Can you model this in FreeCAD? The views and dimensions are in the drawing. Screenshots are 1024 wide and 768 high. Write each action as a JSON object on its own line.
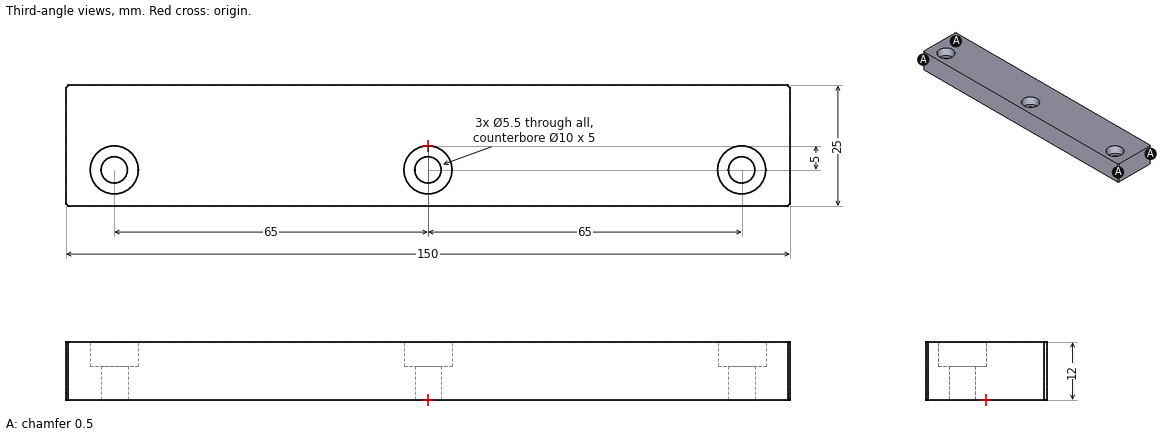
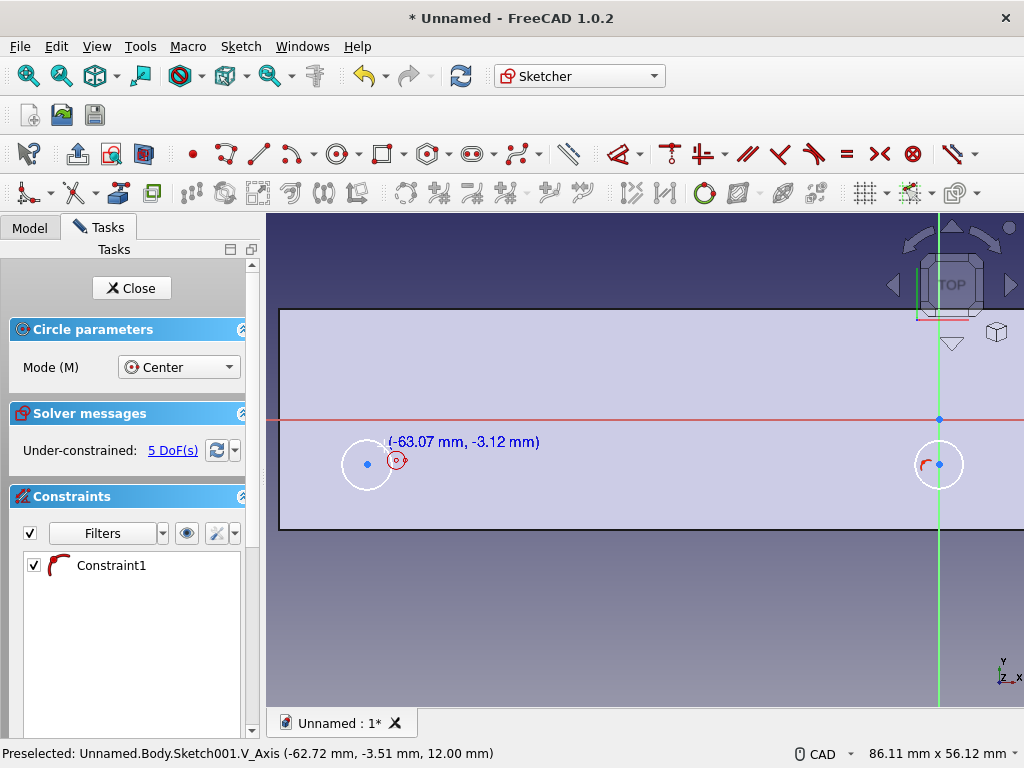
{"action": "scroll", "coordinate": [365, 464], "scroll_direction": "down", "scroll_amount": 5}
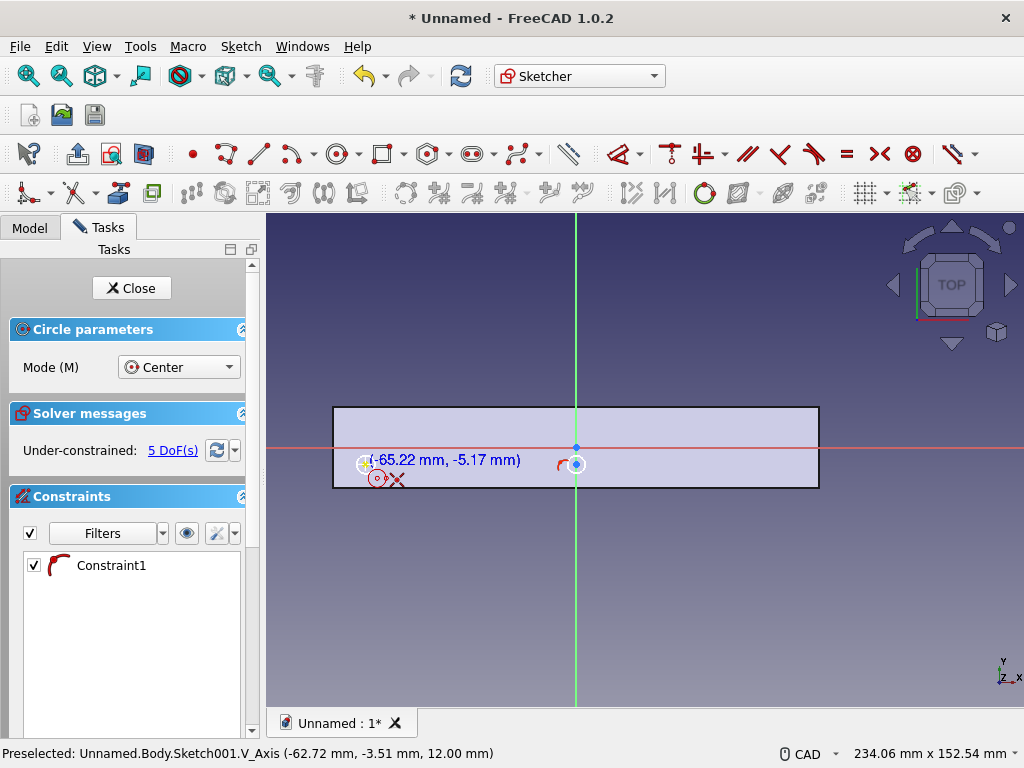
{"action": "scroll", "coordinate": [787, 464], "scroll_direction": "up", "scroll_amount": 5}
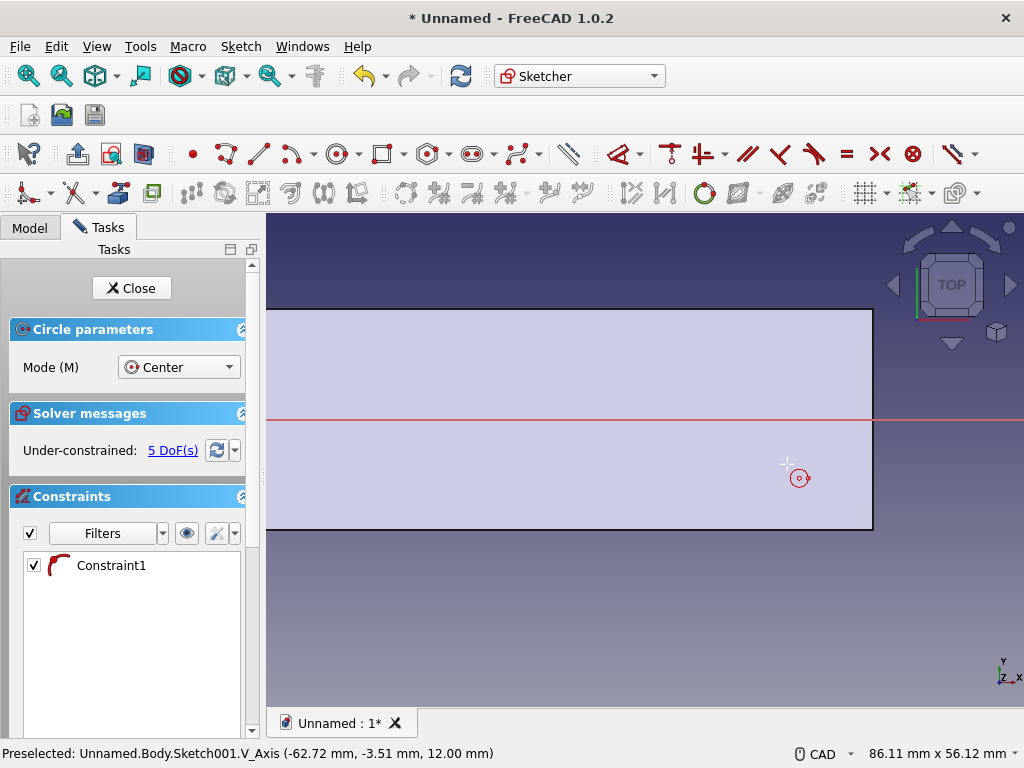
{"action": "left_click", "coordinate": [785, 464]}
{"action": "left_click", "coordinate": [802, 446]}
{"action": "key", "text": "Escape"}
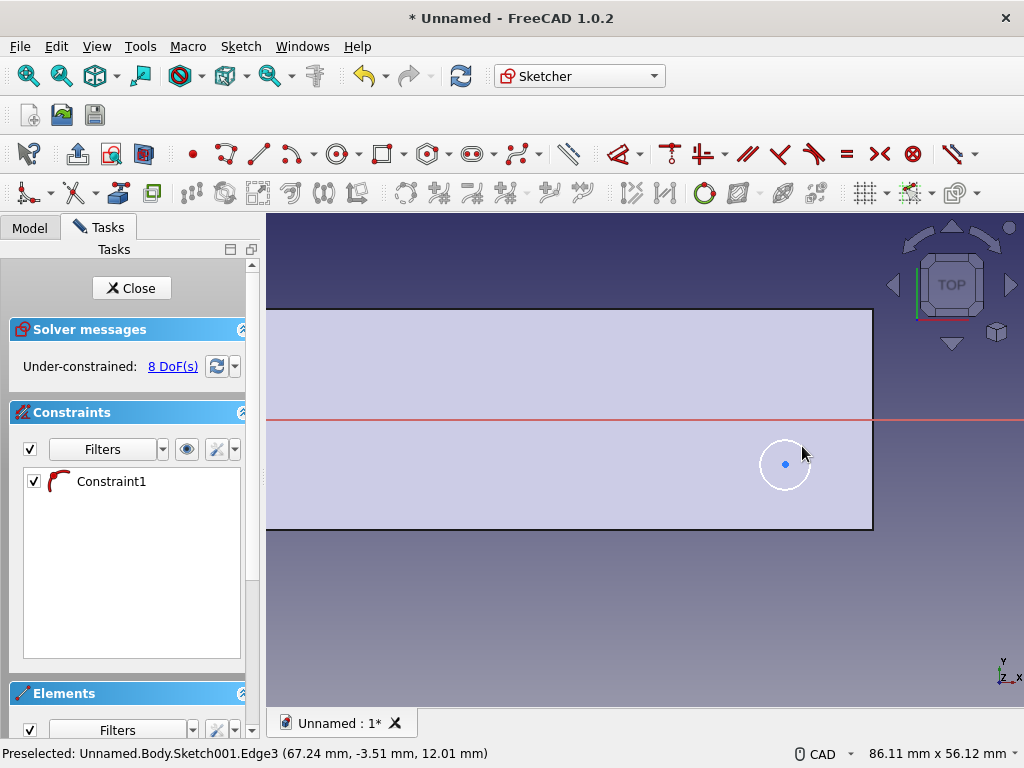
{"action": "scroll", "coordinate": [788, 464], "scroll_direction": "down", "scroll_amount": 5}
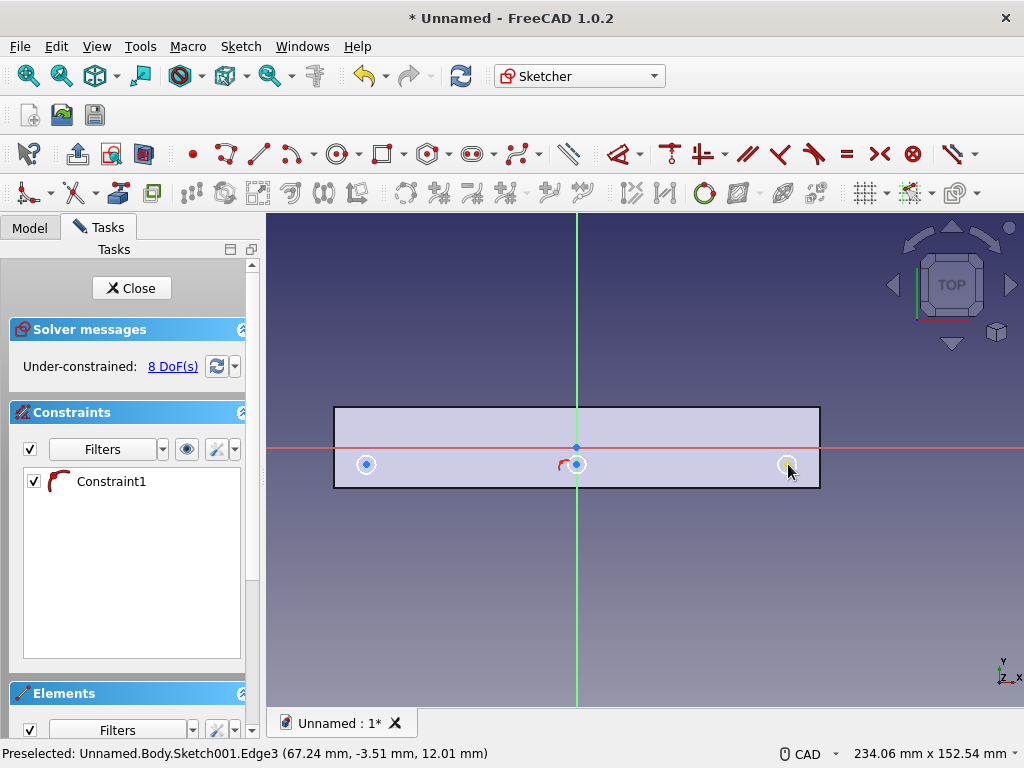
{"action": "scroll", "coordinate": [583, 458], "scroll_direction": "up", "scroll_amount": 5}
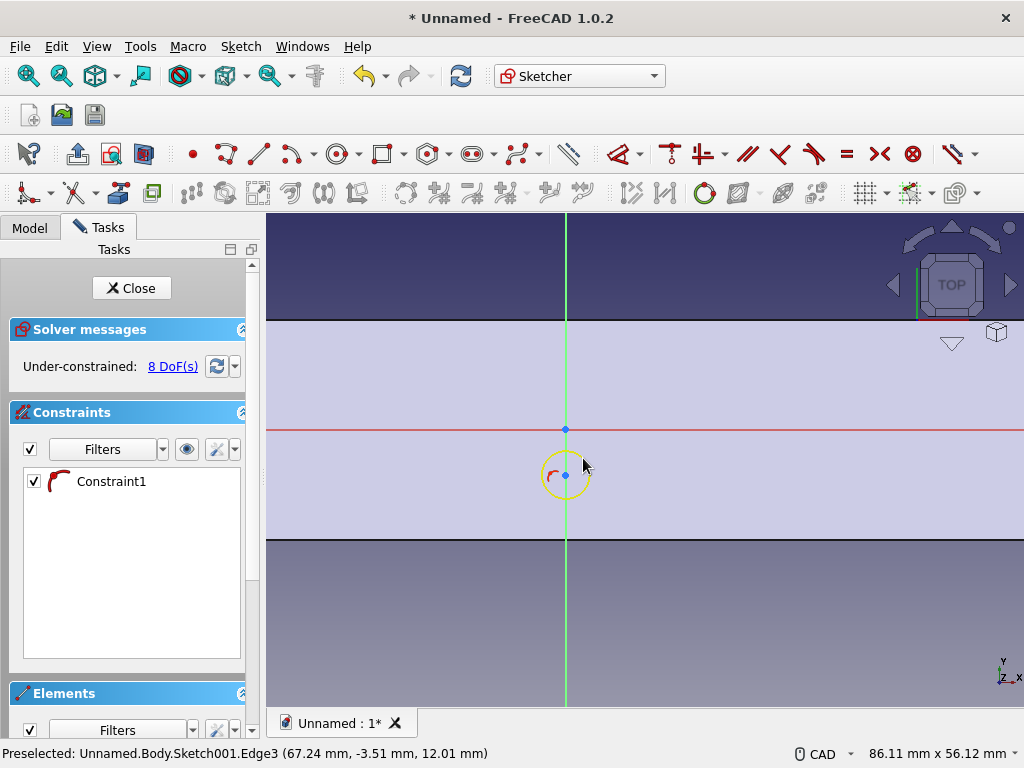
{"action": "left_click", "coordinate": [583, 458]}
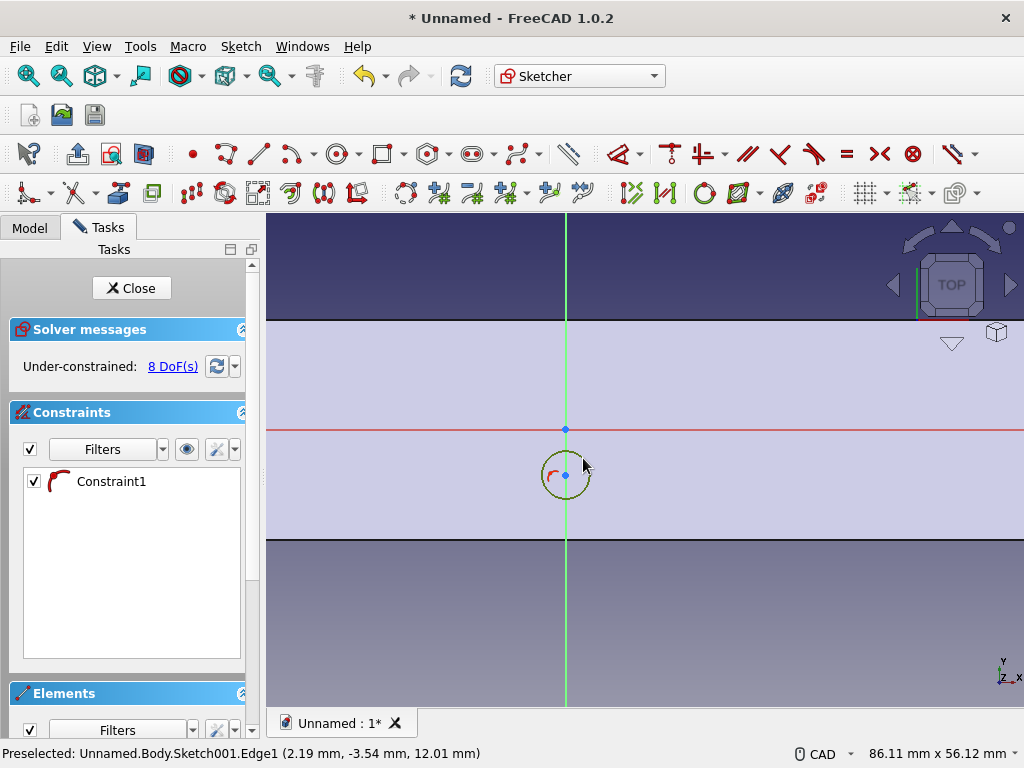
{"action": "scroll", "coordinate": [583, 458], "scroll_direction": "down", "scroll_amount": 5}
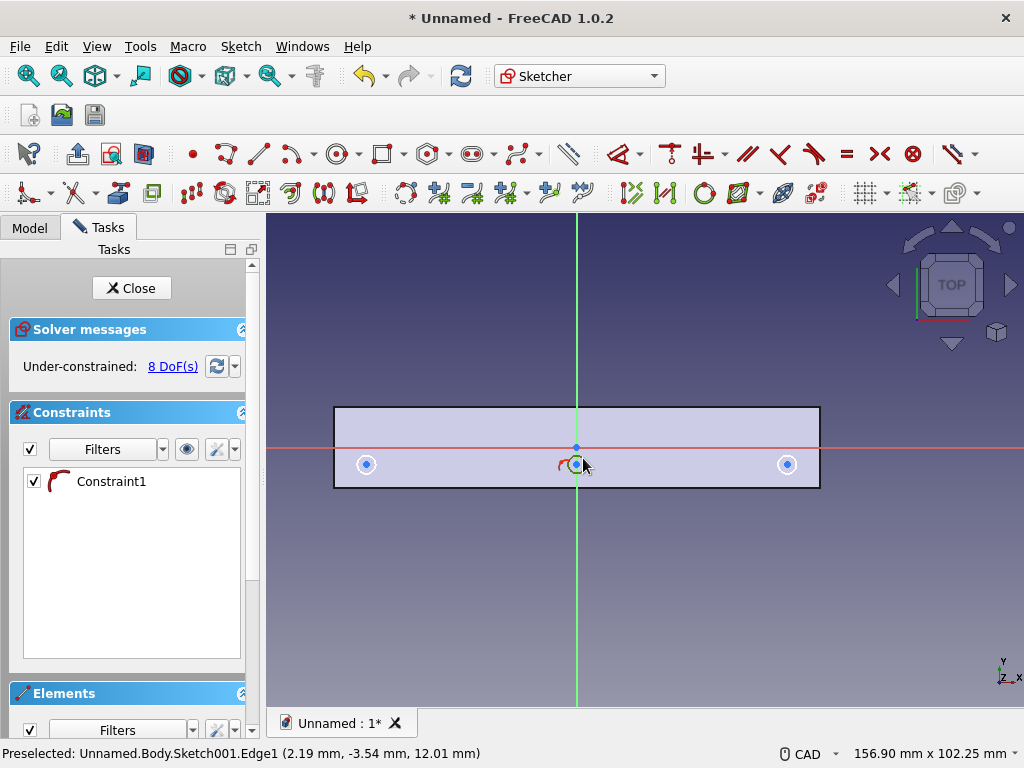
{"action": "scroll", "coordinate": [373, 458], "scroll_direction": "up", "scroll_amount": 3}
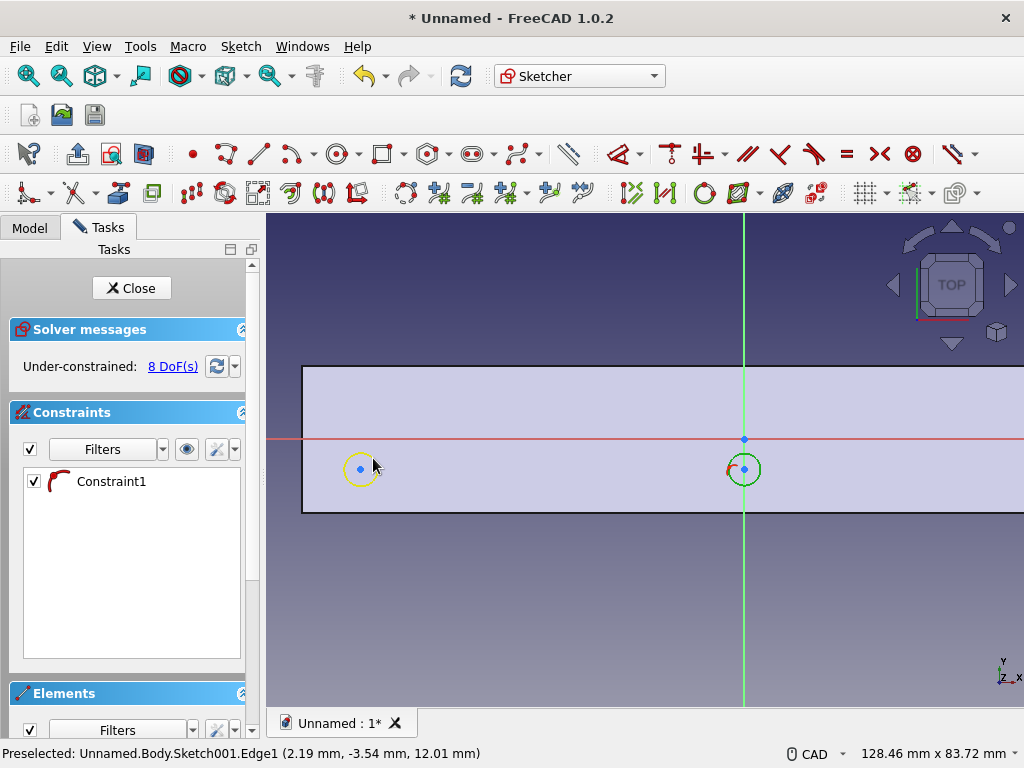
{"action": "left_click", "coordinate": [373, 458]}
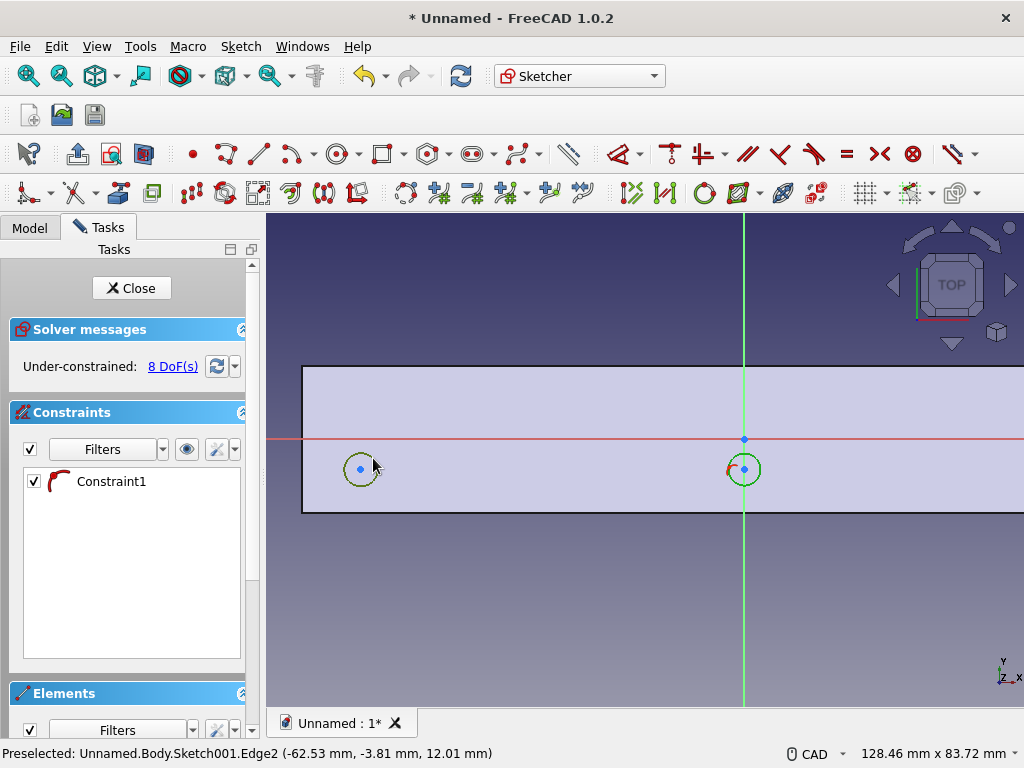
{"action": "scroll", "coordinate": [372, 457], "scroll_direction": "down", "scroll_amount": 3}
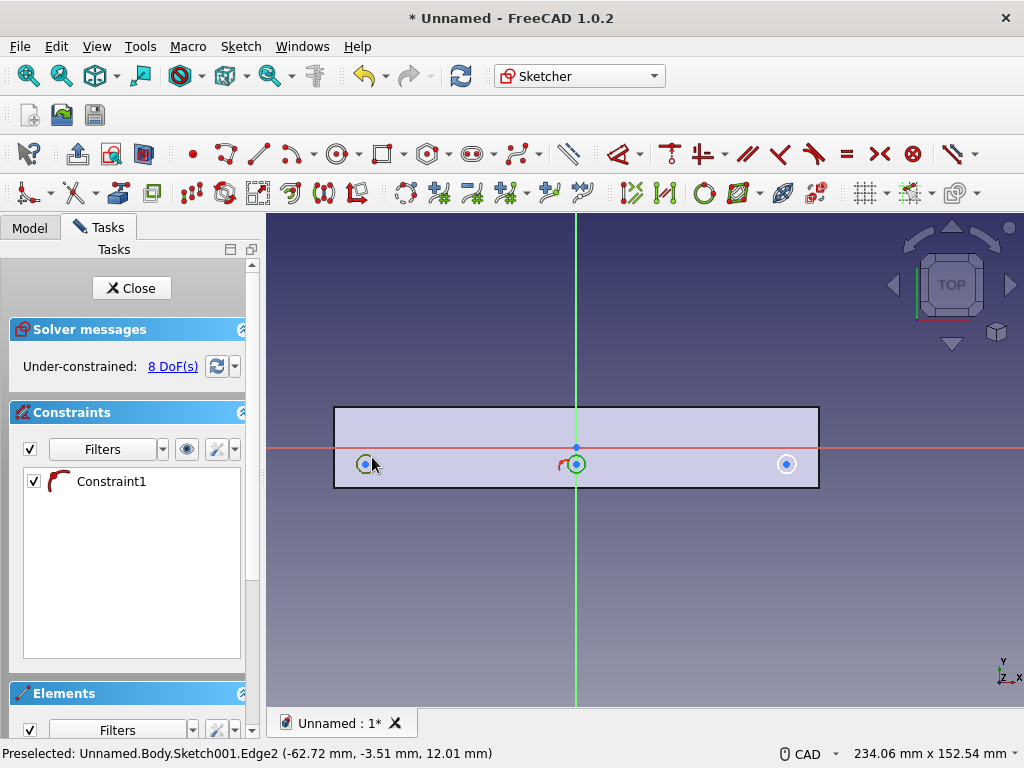
{"action": "scroll", "coordinate": [793, 458], "scroll_direction": "up", "scroll_amount": 3}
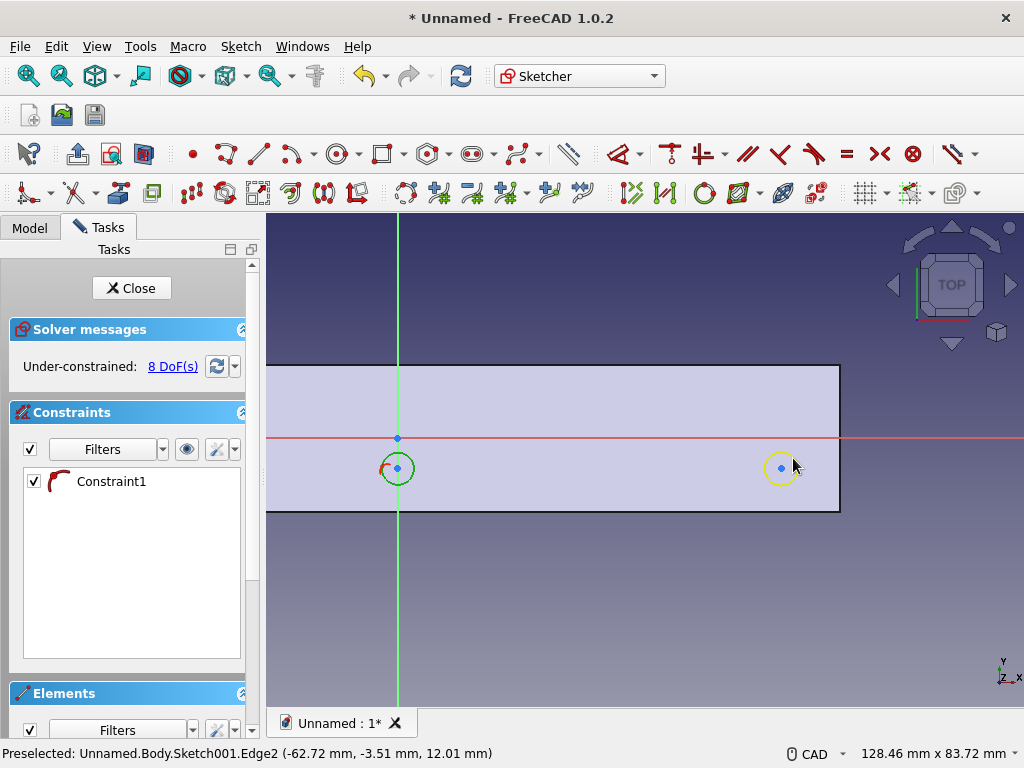
{"action": "left_click", "coordinate": [793, 457]}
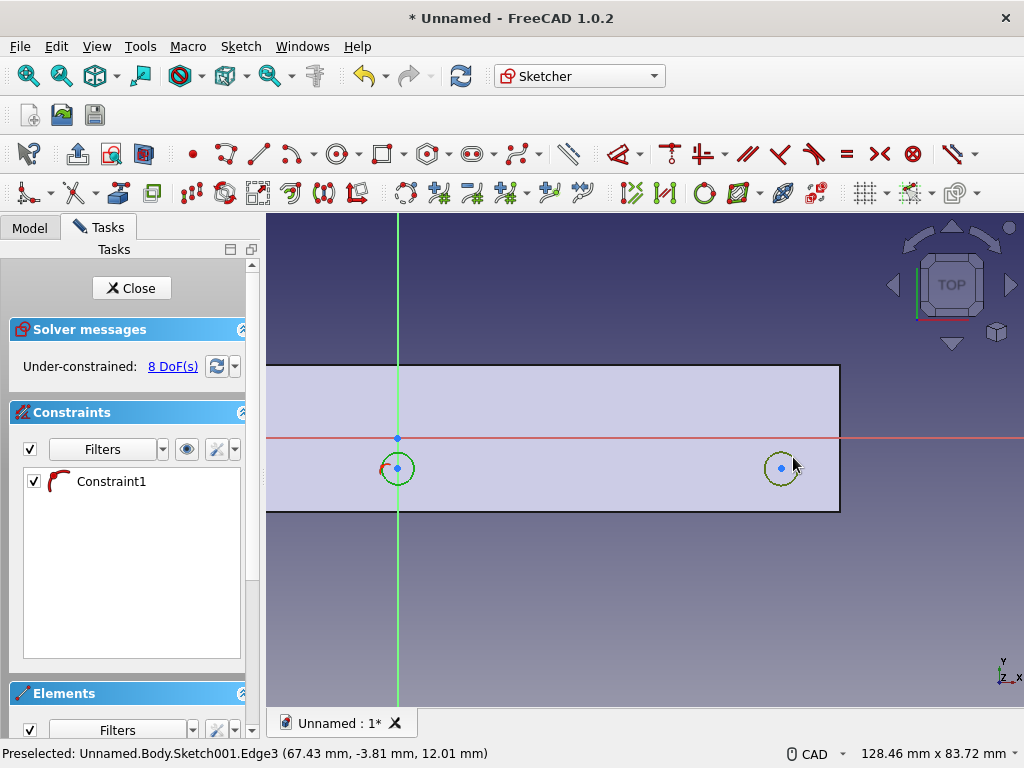
{"action": "left_click", "coordinate": [847, 154]}